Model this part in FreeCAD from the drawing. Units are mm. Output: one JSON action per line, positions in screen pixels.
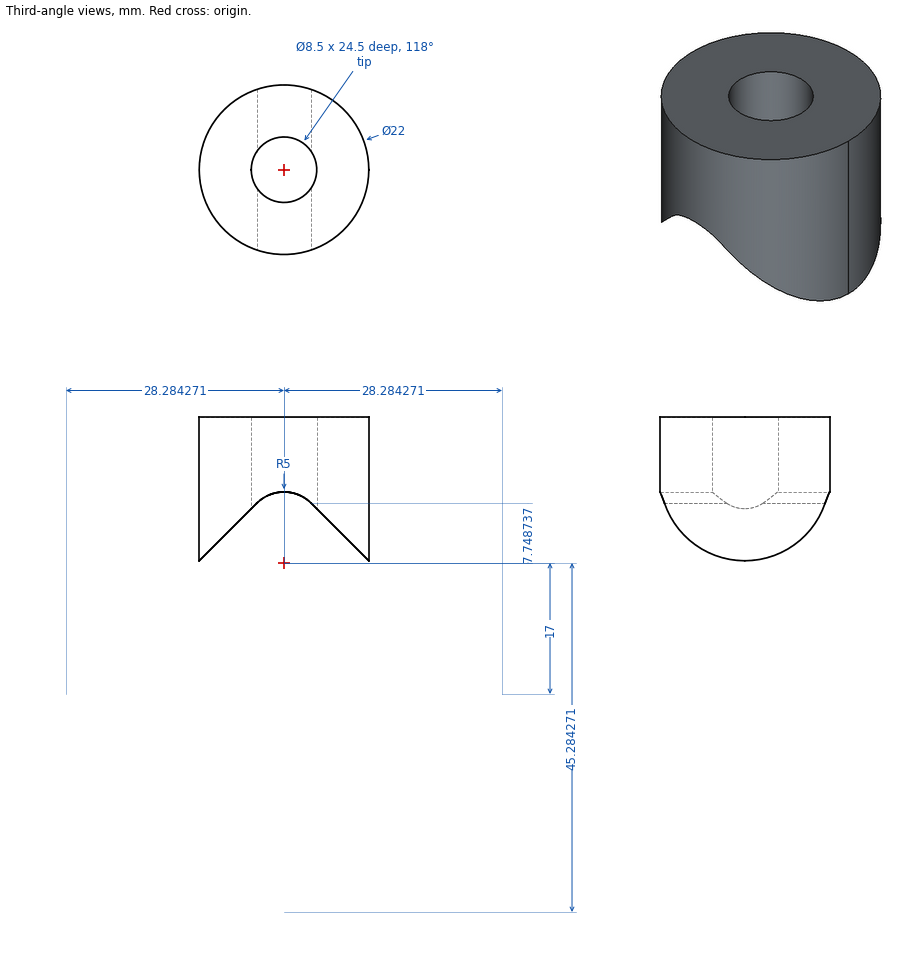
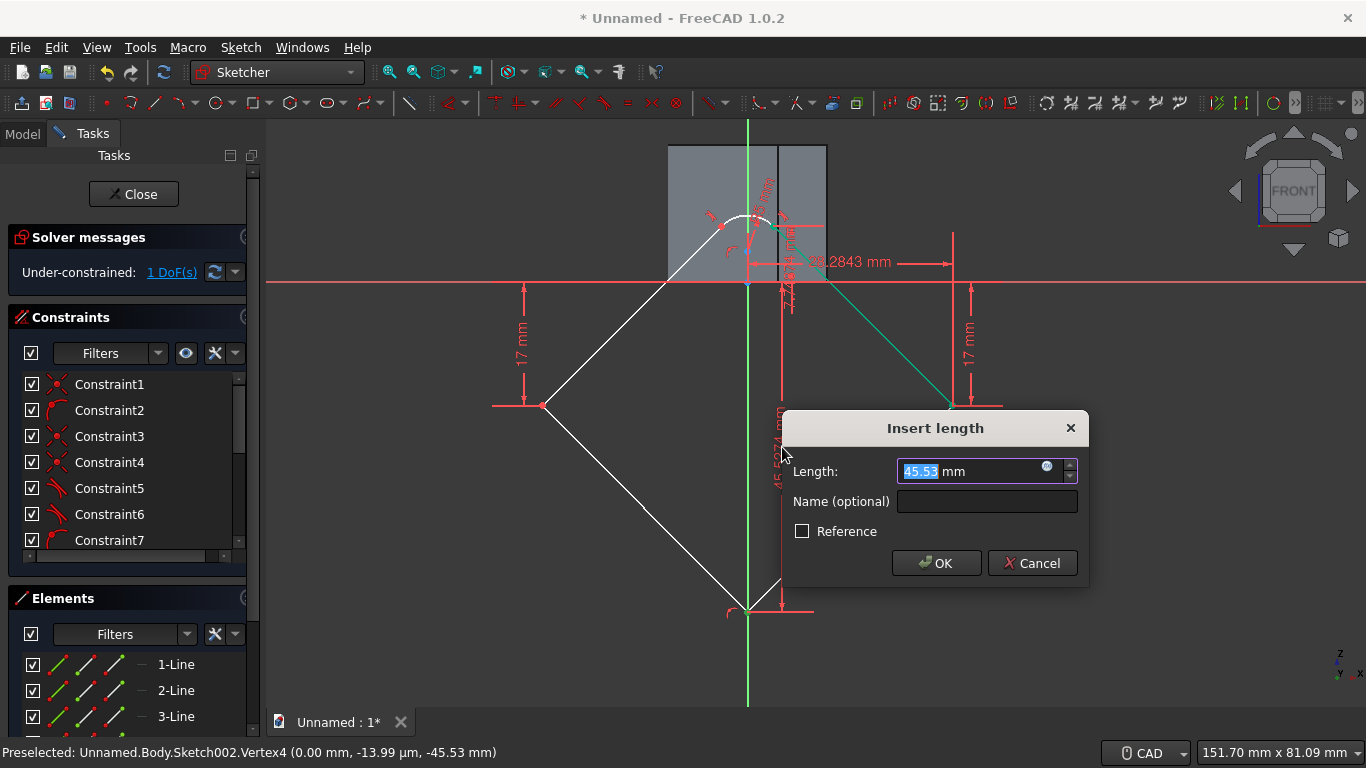
{"action": "type", "text": "45.284271"}
{"action": "key", "text": "Return"}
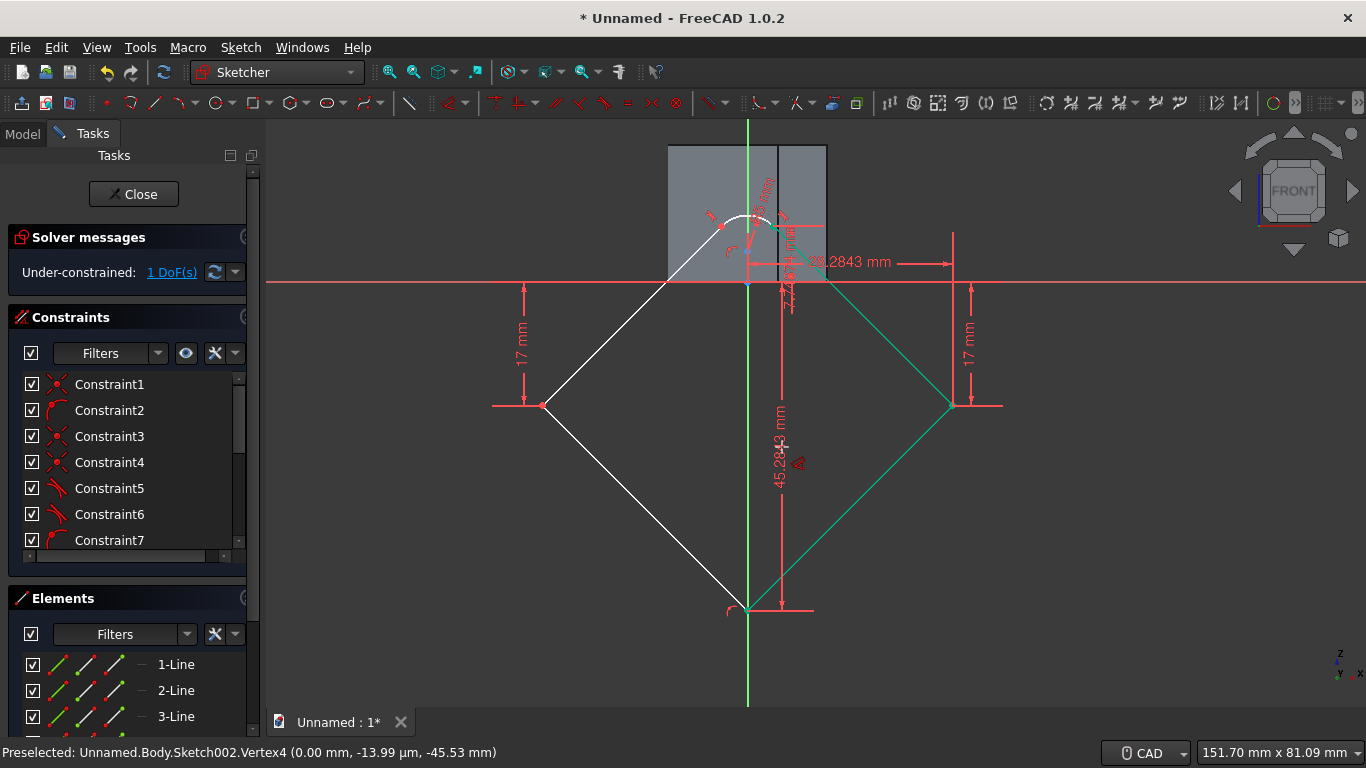
{"action": "left_click", "coordinate": [542, 406]}
{"action": "left_click", "coordinate": [645, 248]}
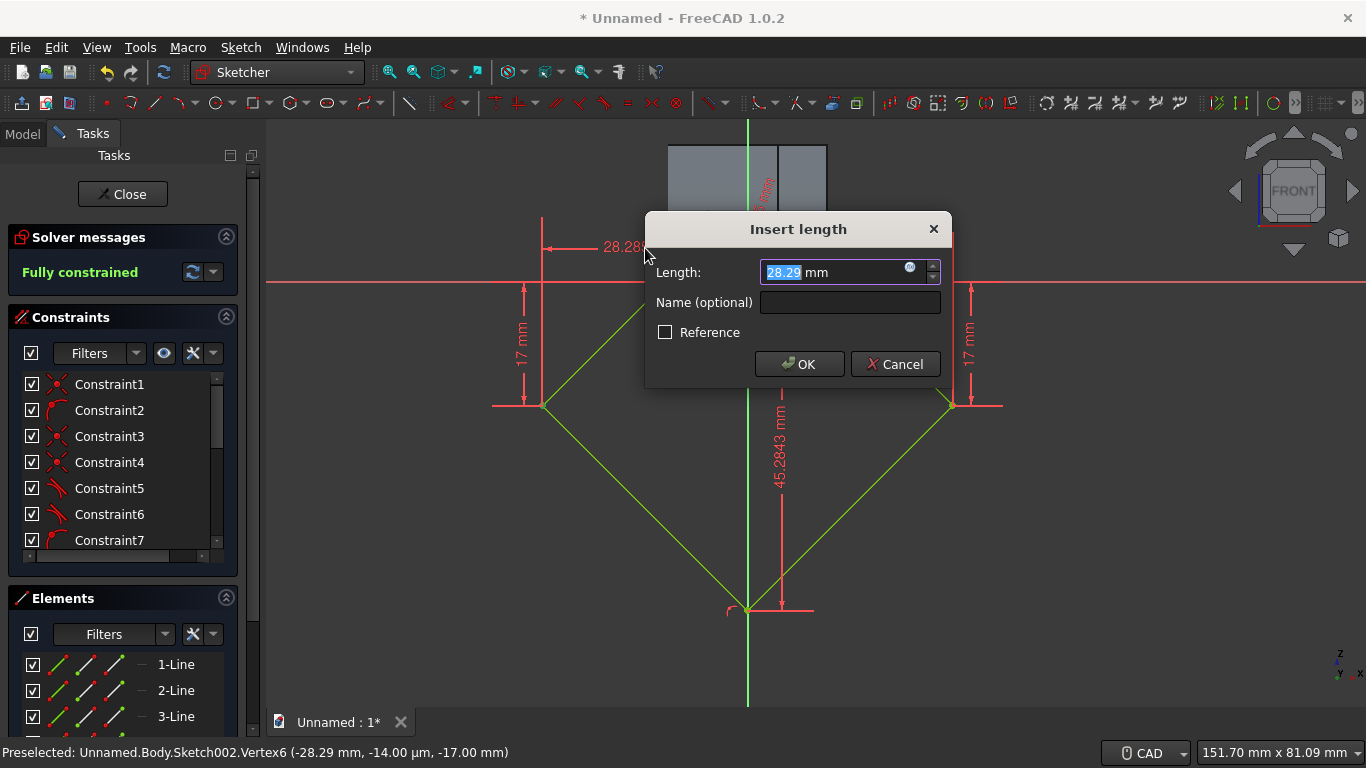
{"action": "type", "text": "28.284271"}
{"action": "key", "text": "Return"}
{"action": "key", "text": "Escape"}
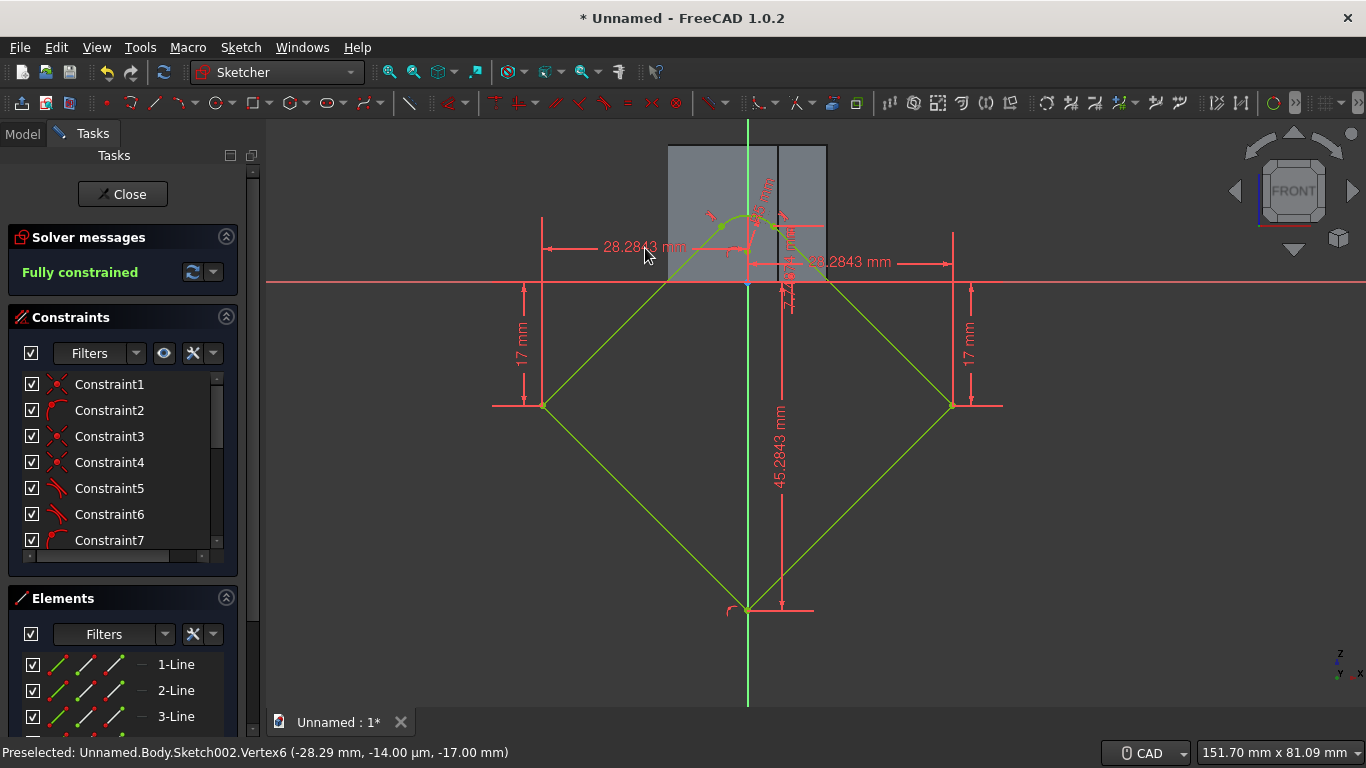
{"action": "left_click", "coordinate": [123, 194]}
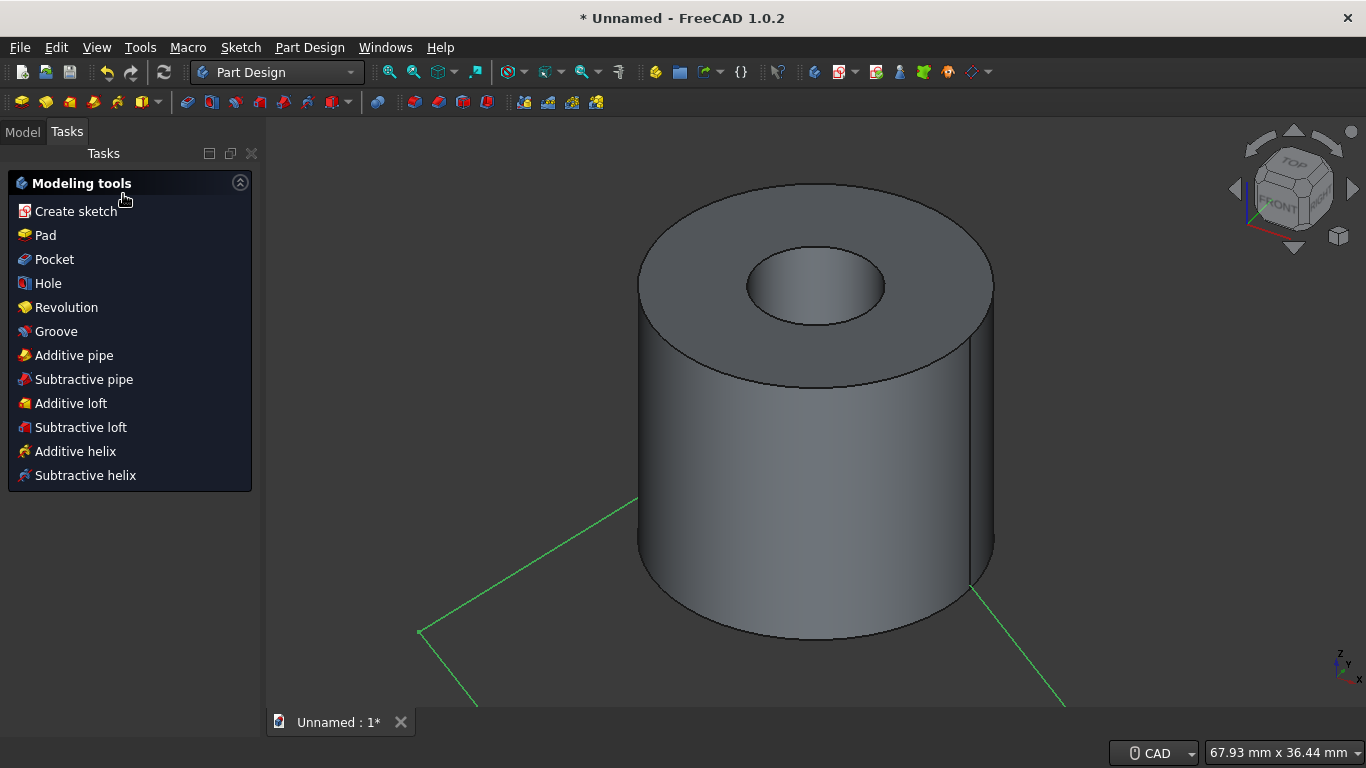
{"action": "left_click", "coordinate": [188, 102]}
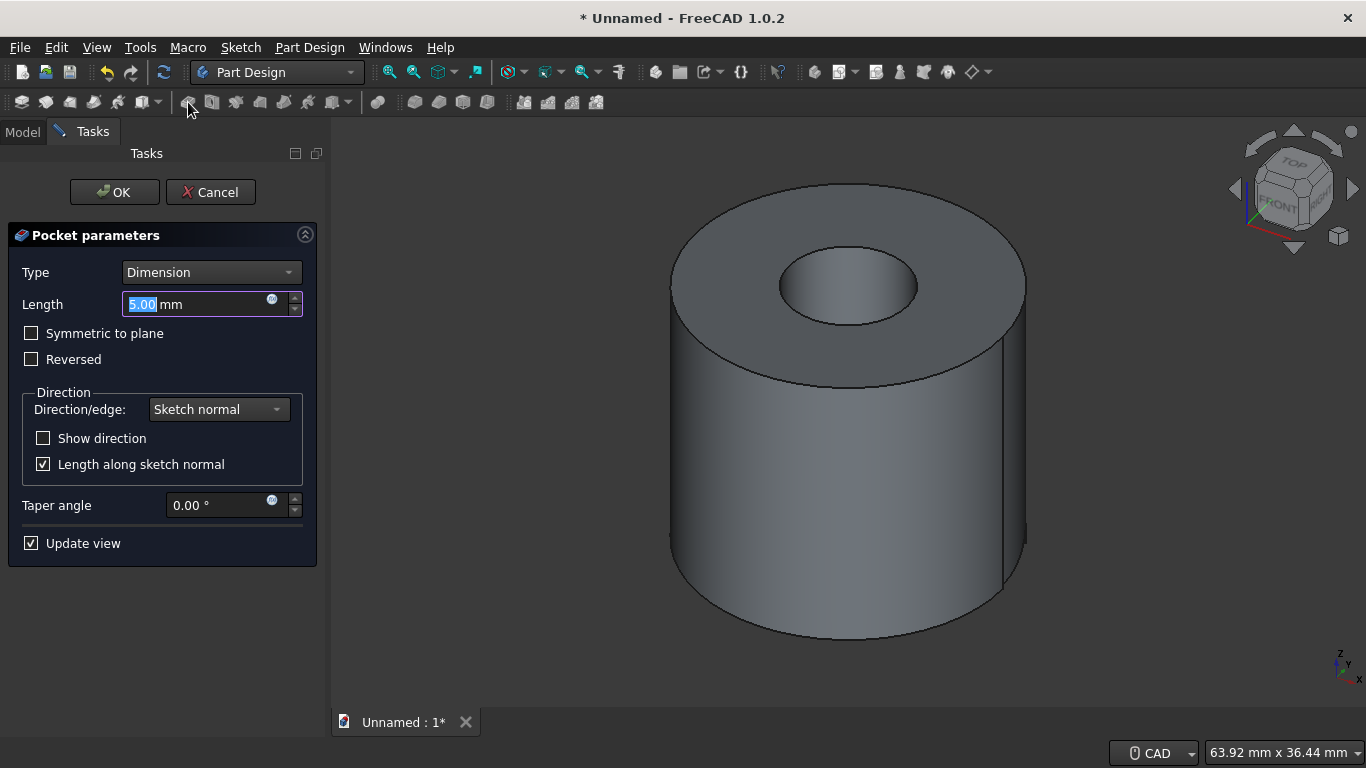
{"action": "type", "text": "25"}
{"action": "key", "text": "Tab"}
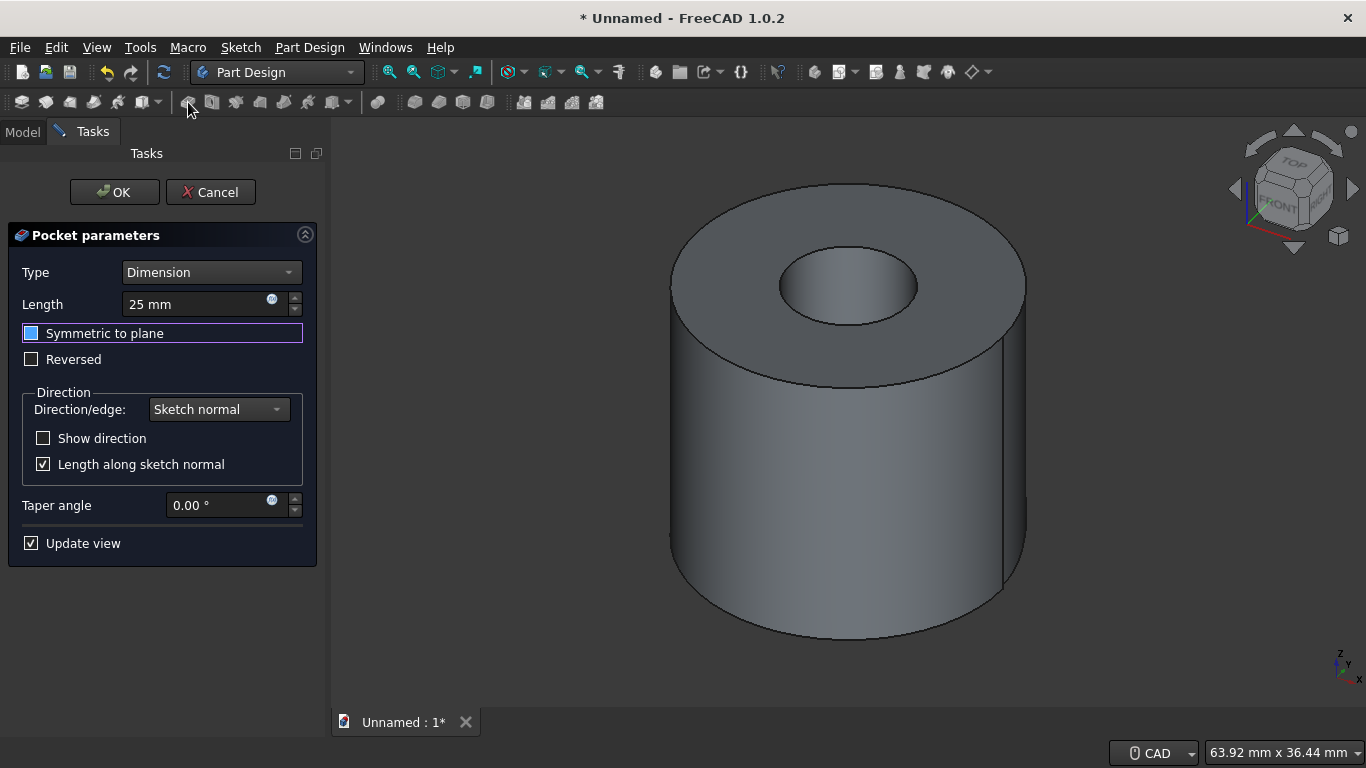
{"action": "left_click", "coordinate": [30, 333]}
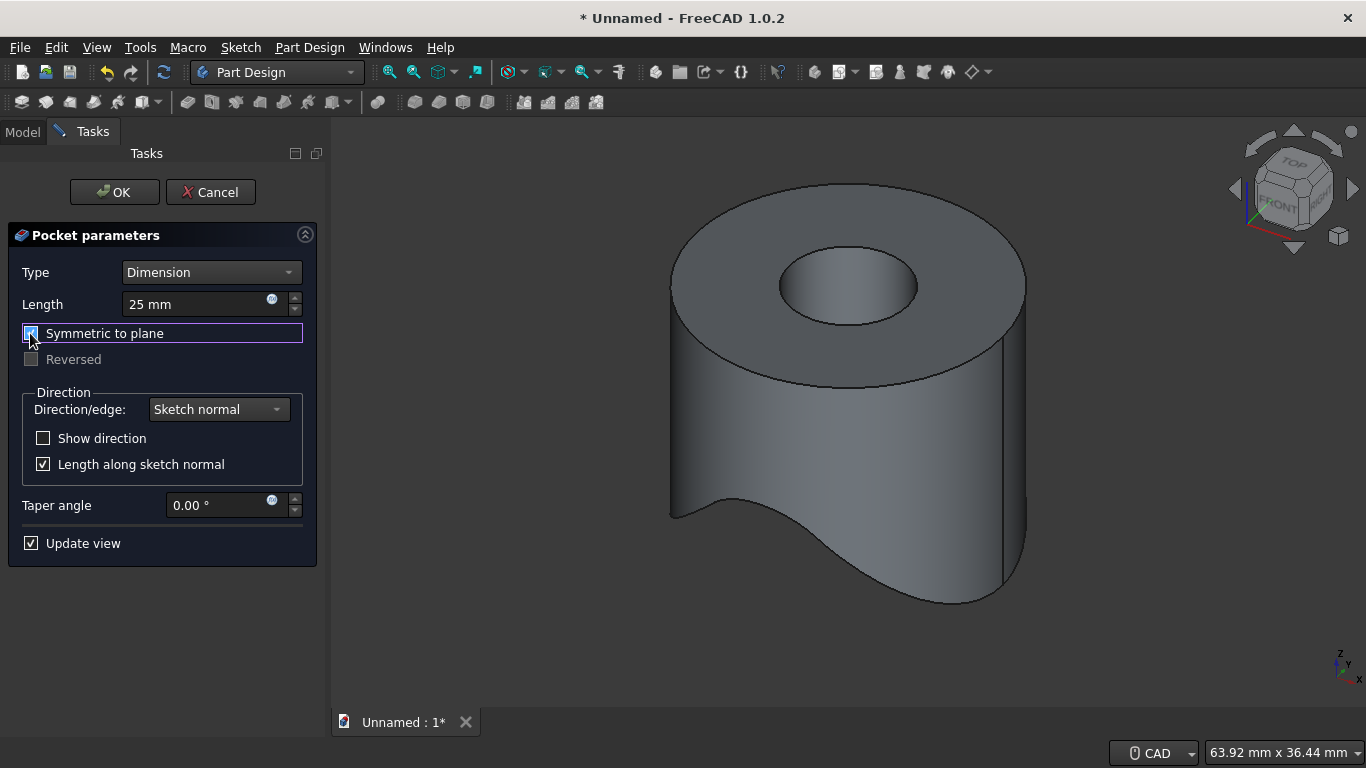
{"action": "left_click", "coordinate": [115, 192]}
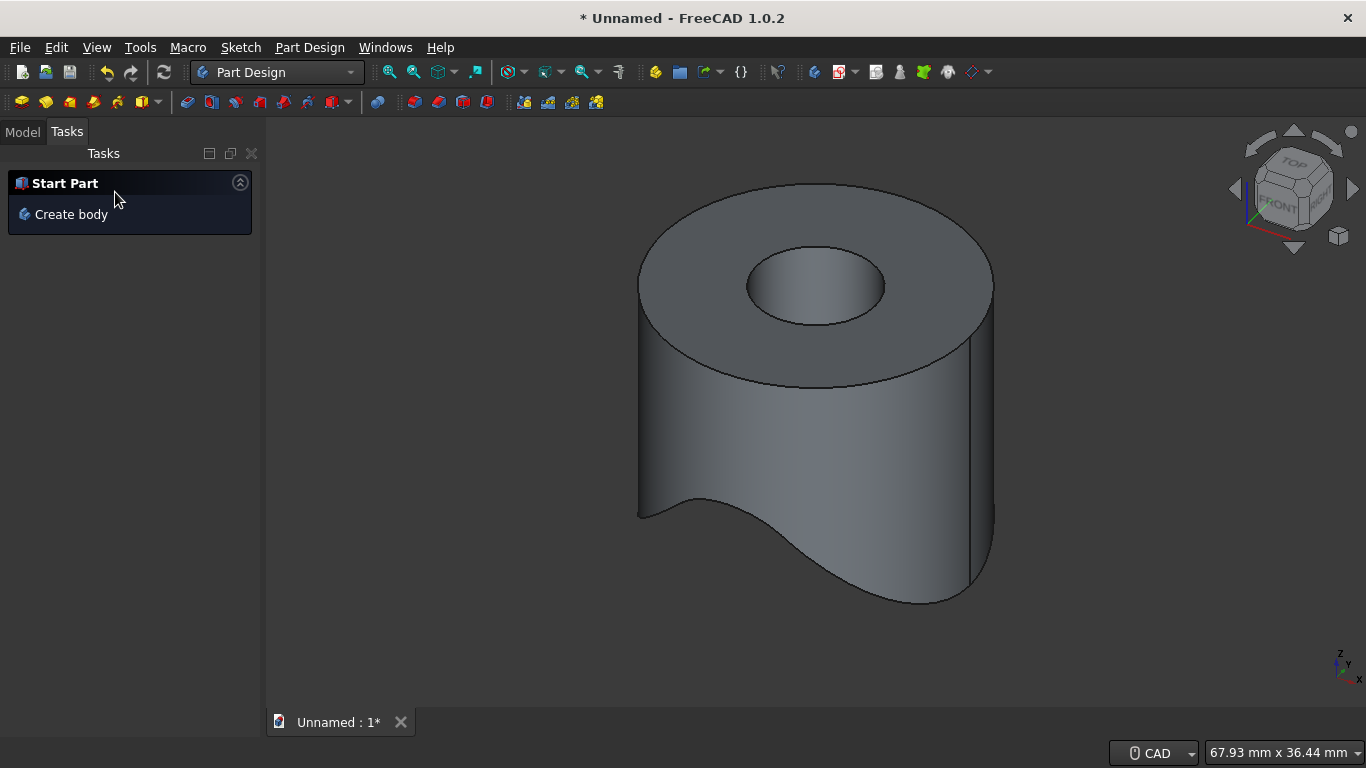
{"action": "key", "text": "0"}